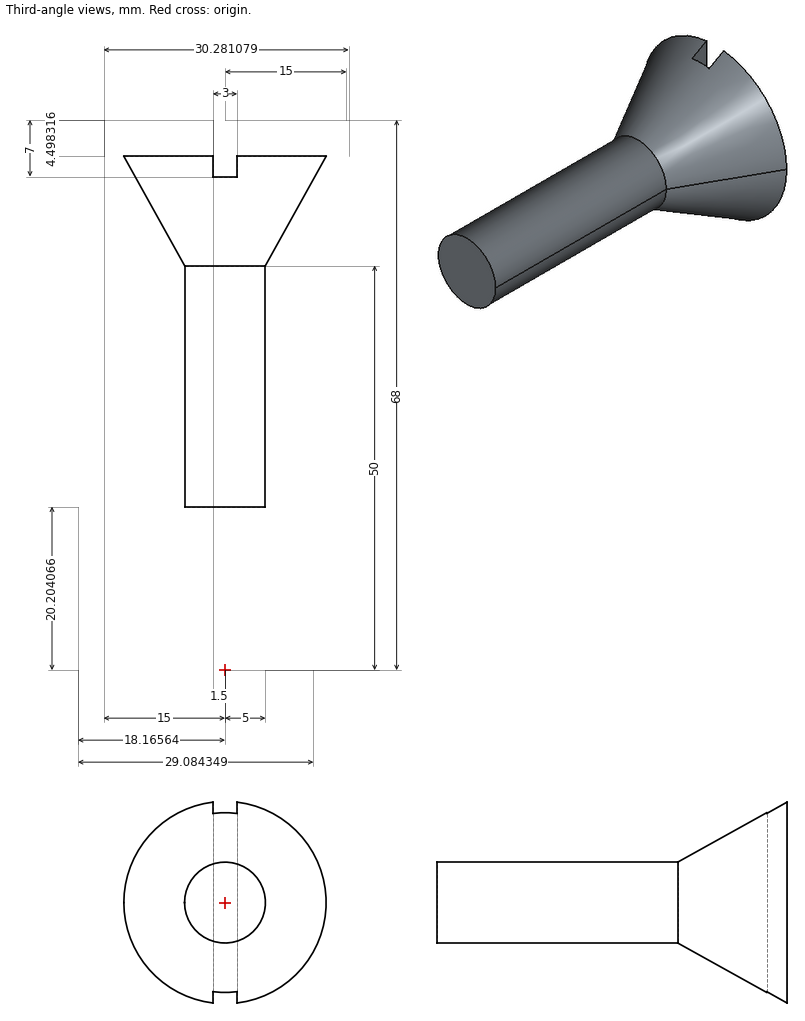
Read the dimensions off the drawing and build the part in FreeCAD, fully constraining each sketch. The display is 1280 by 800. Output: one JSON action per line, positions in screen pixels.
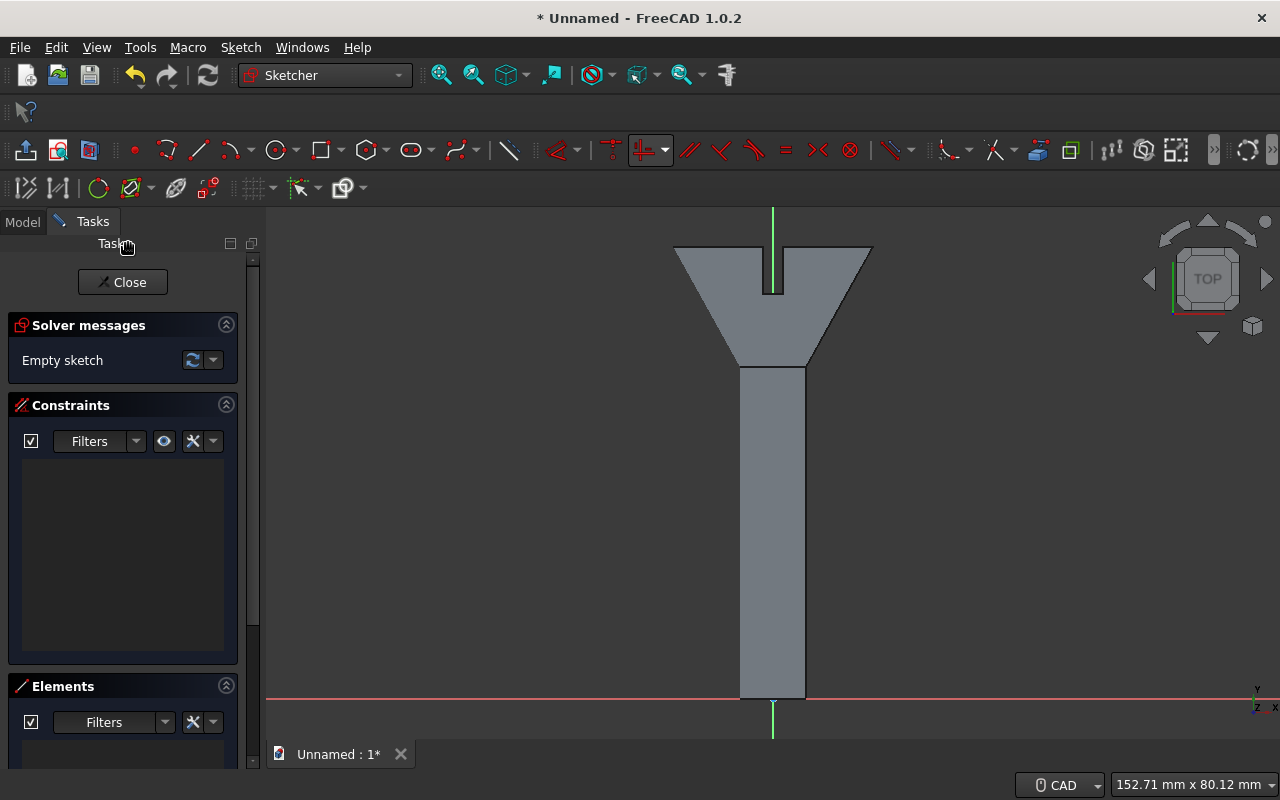
{"action": "left_click", "coordinate": [90, 150]}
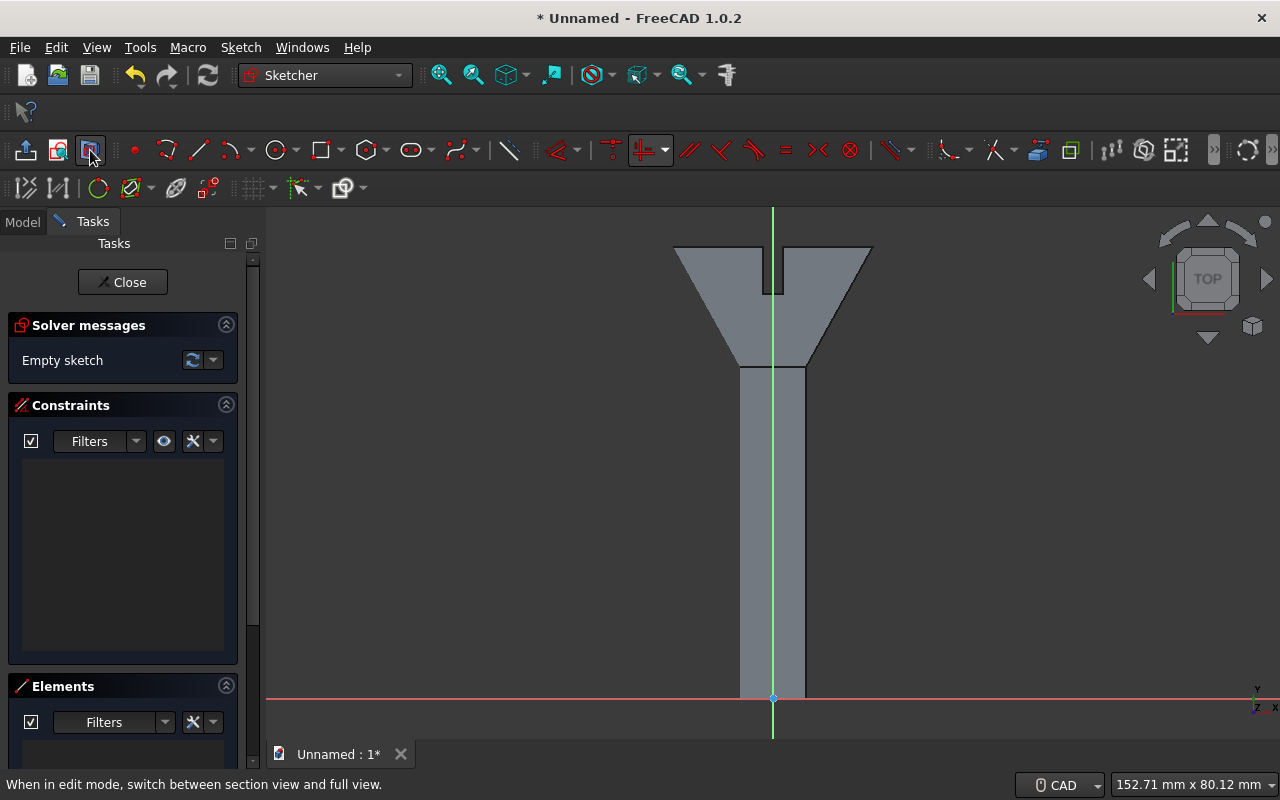
{"action": "scroll", "coordinate": [391, 473], "scroll_direction": "down", "scroll_amount": 1}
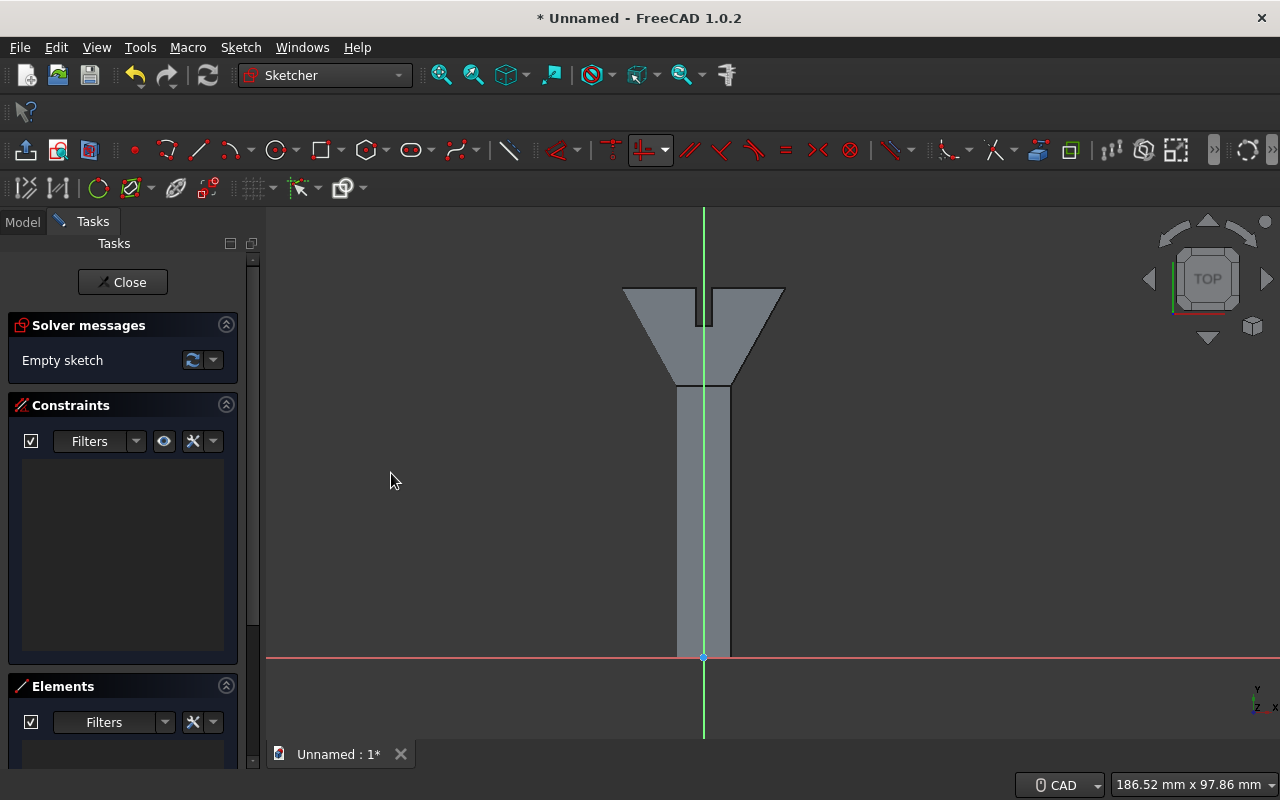
{"action": "left_click", "coordinate": [322, 150]}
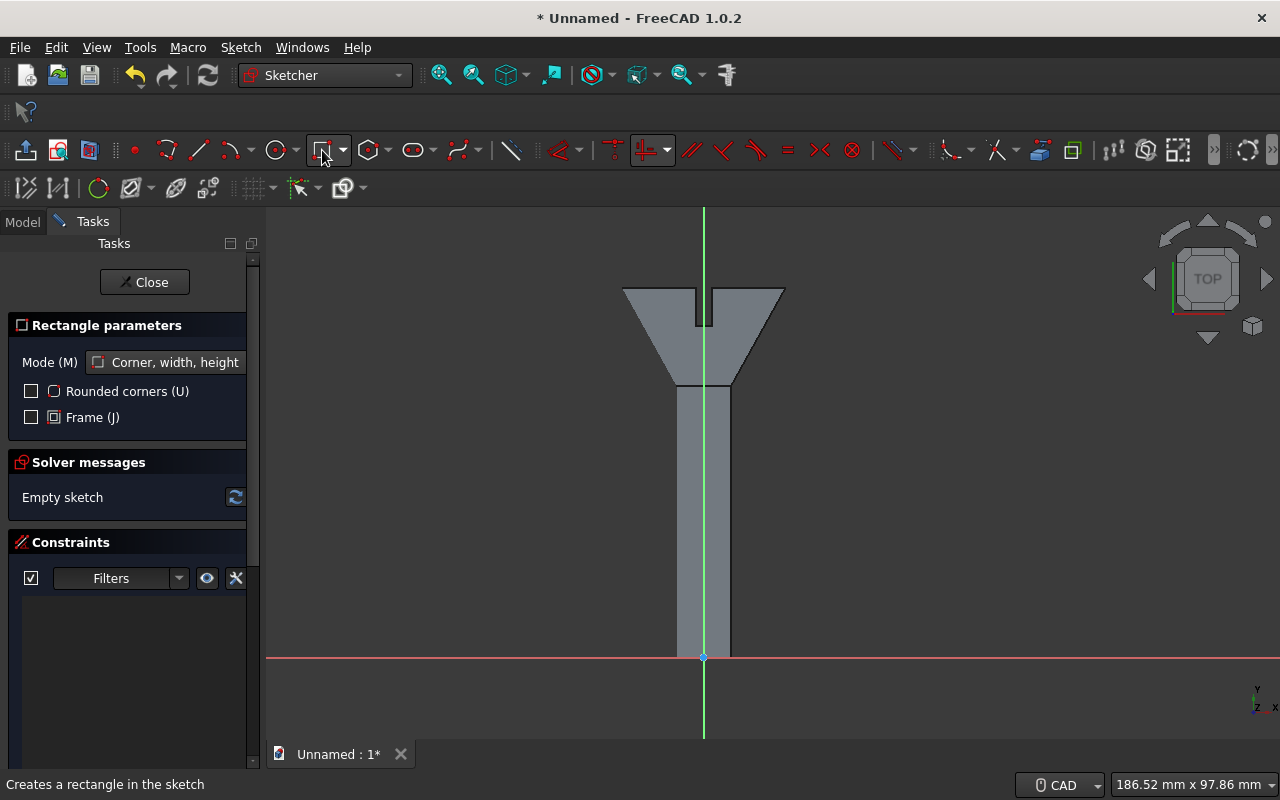
{"action": "left_click", "coordinate": [622, 288]}
{"action": "left_click", "coordinate": [787, 313]}
{"action": "key", "text": "Escape"}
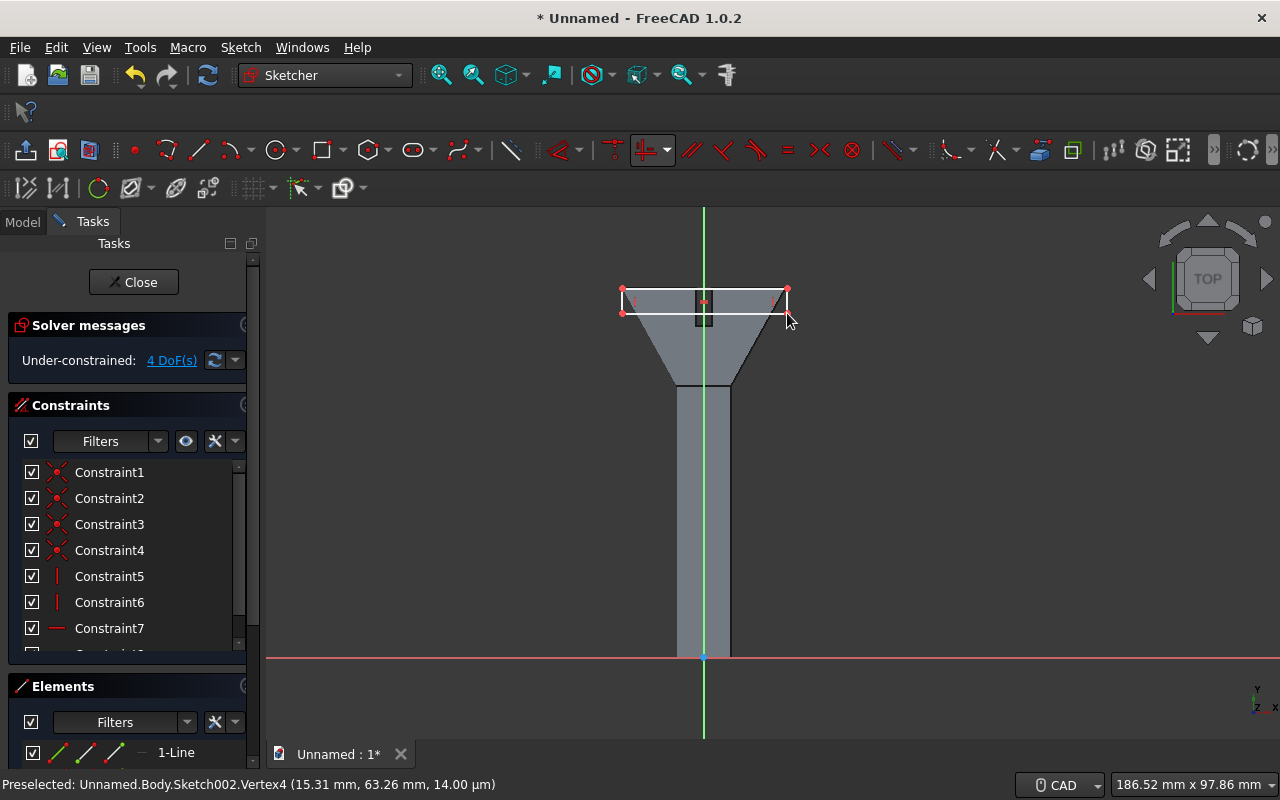
{"action": "left_click", "coordinate": [558, 150]}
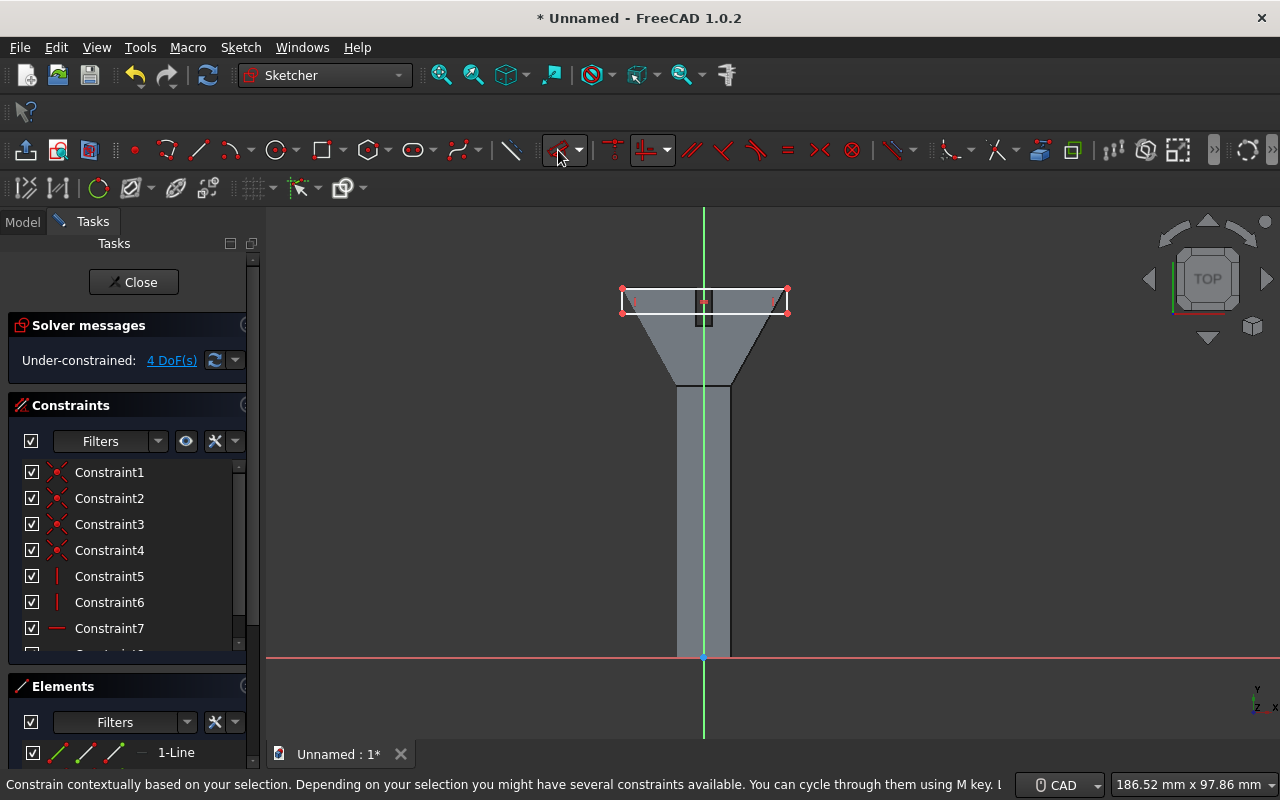
{"action": "left_click", "coordinate": [622, 289]}
{"action": "left_click", "coordinate": [663, 692]}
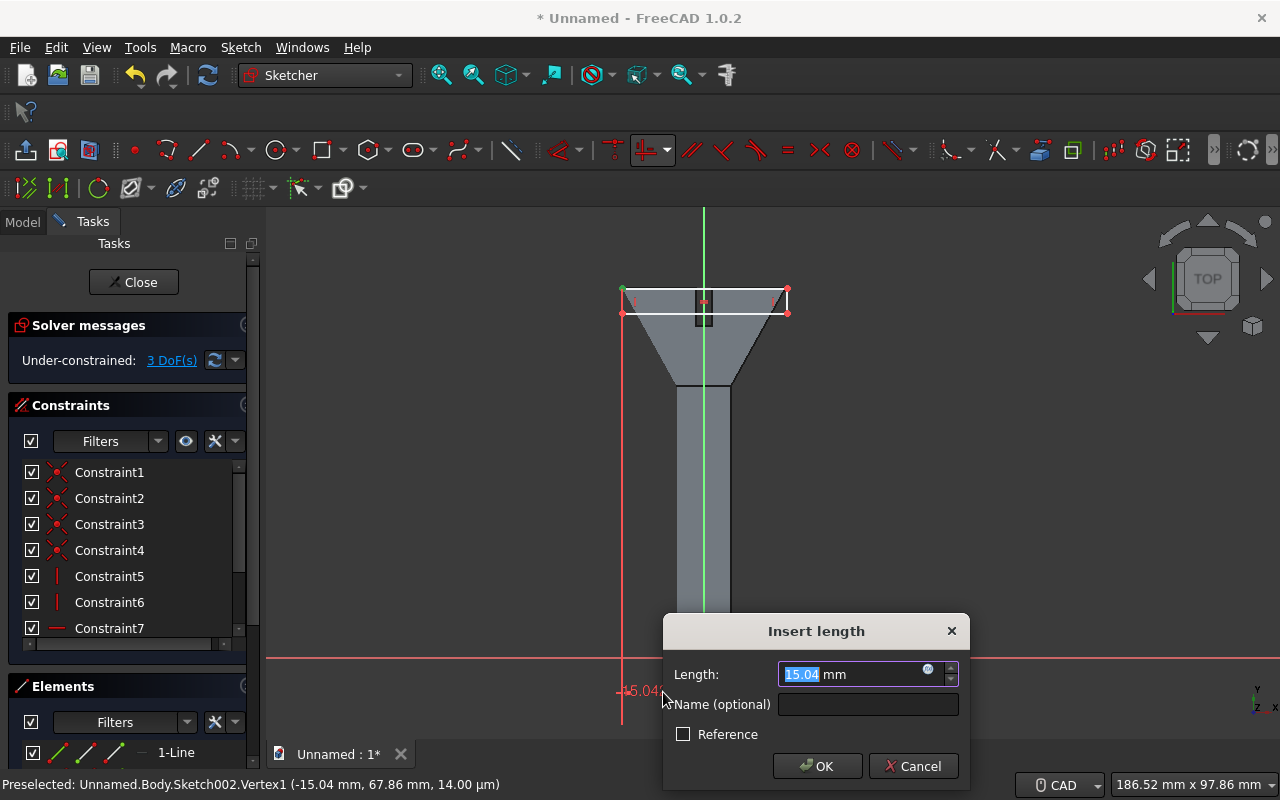
{"action": "type", "text": "15"}
{"action": "key", "text": "Return"}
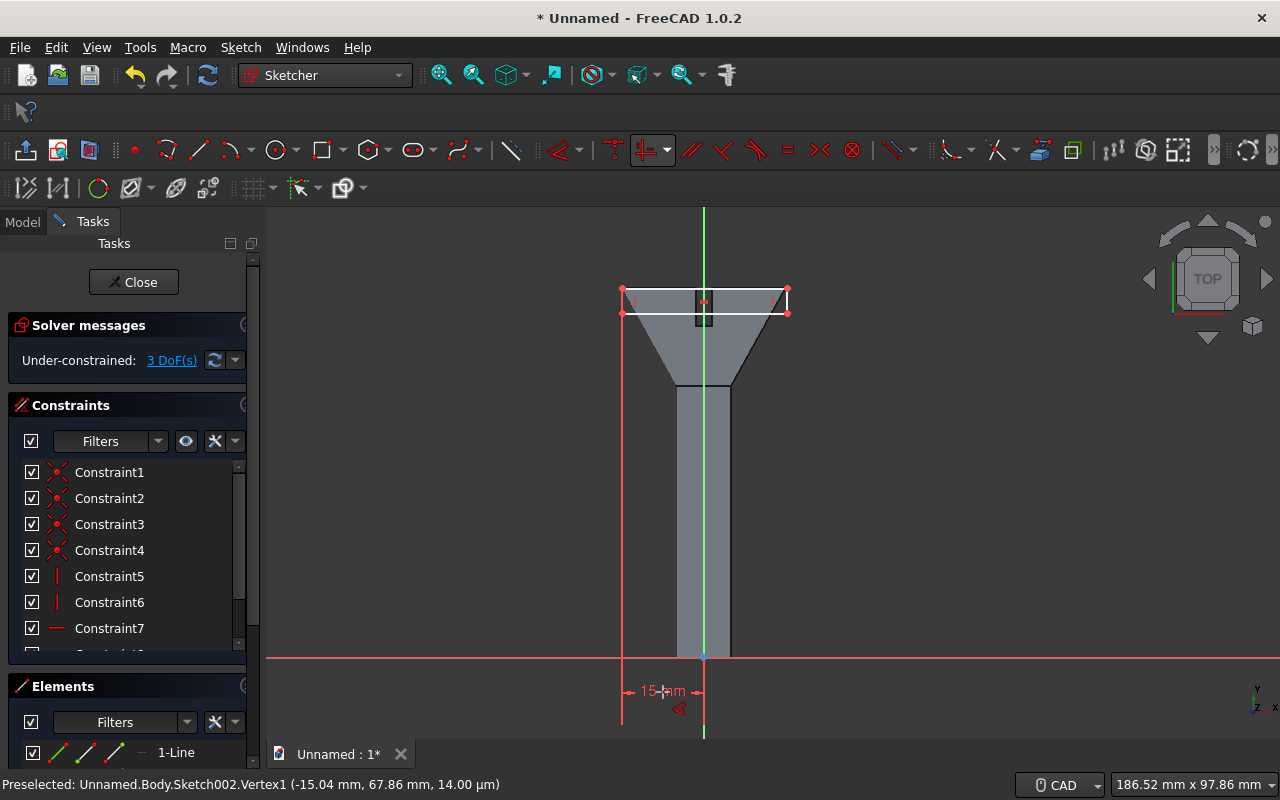
{"action": "left_click", "coordinate": [622, 289]}
{"action": "left_click", "coordinate": [588, 473]}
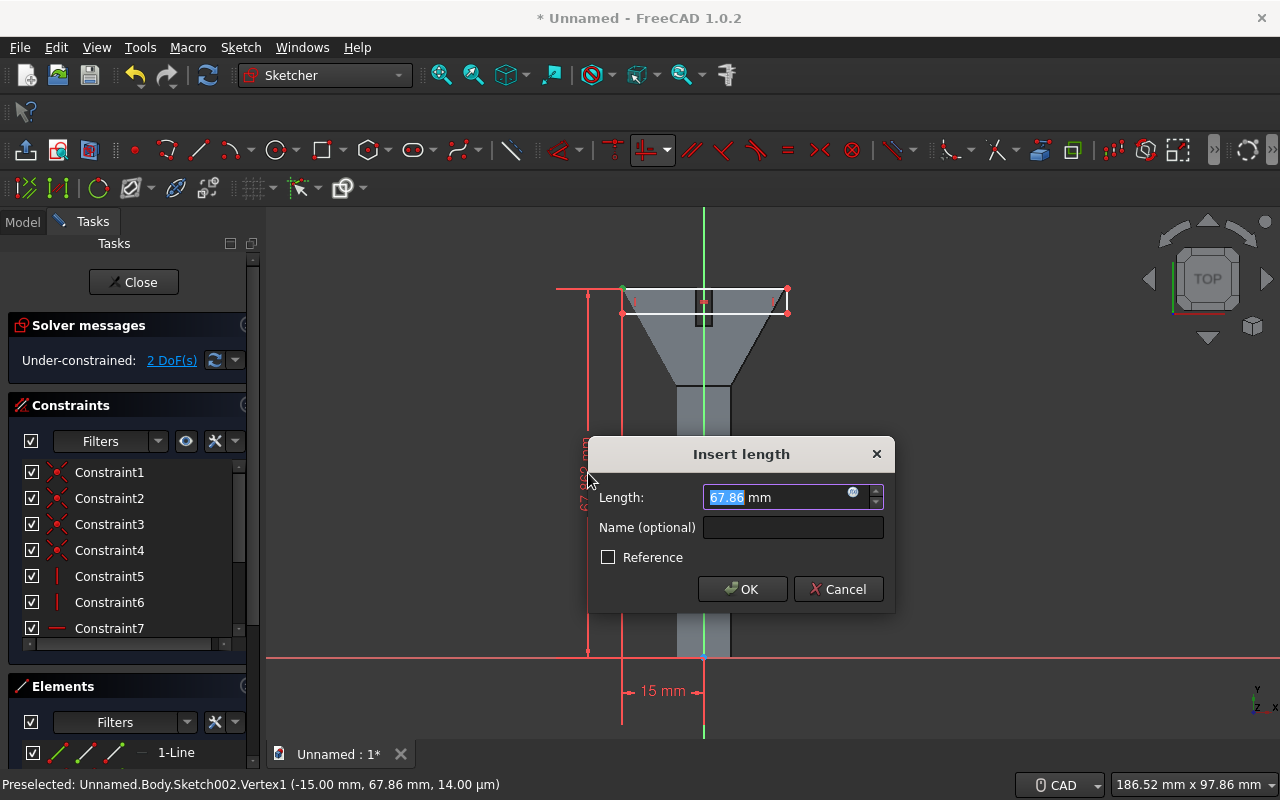
{"action": "type", "text": "68"}
{"action": "key", "text": "Return"}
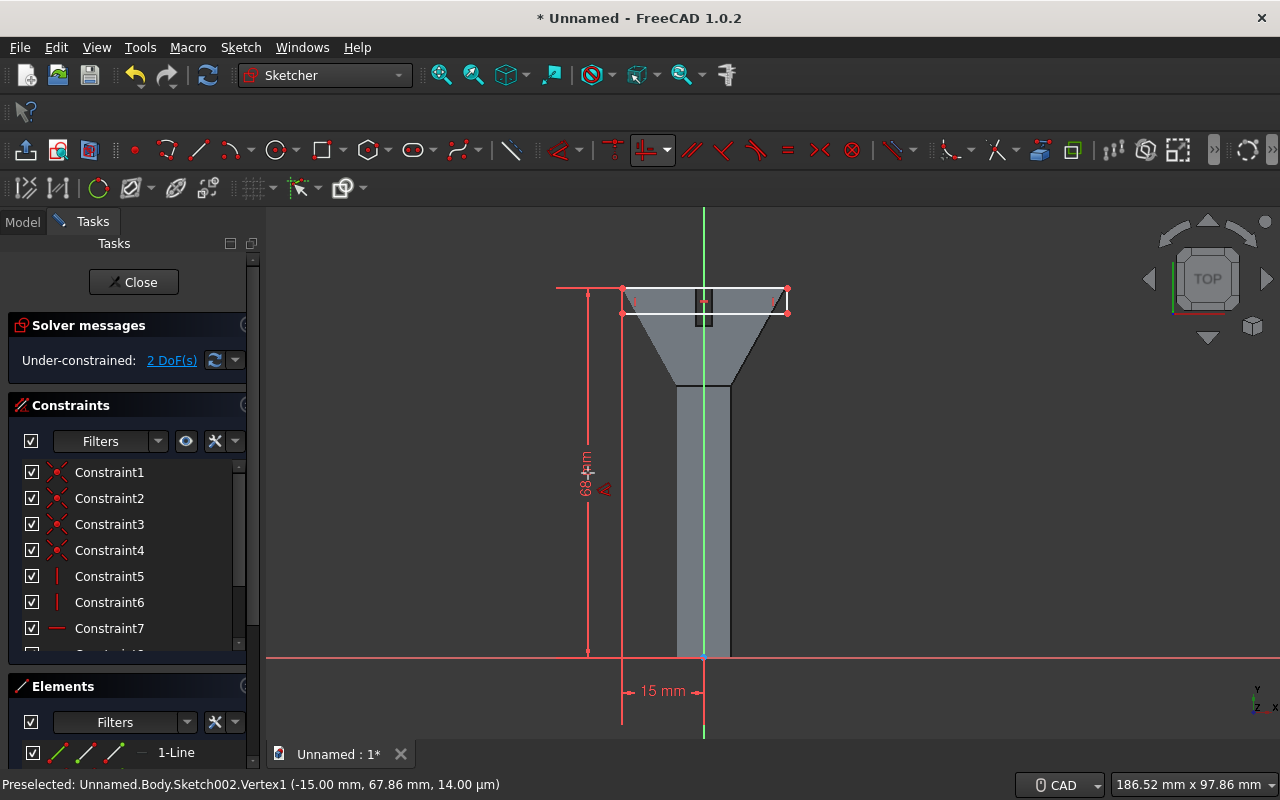
{"action": "scroll", "coordinate": [622, 299], "scroll_direction": "up", "scroll_amount": 3}